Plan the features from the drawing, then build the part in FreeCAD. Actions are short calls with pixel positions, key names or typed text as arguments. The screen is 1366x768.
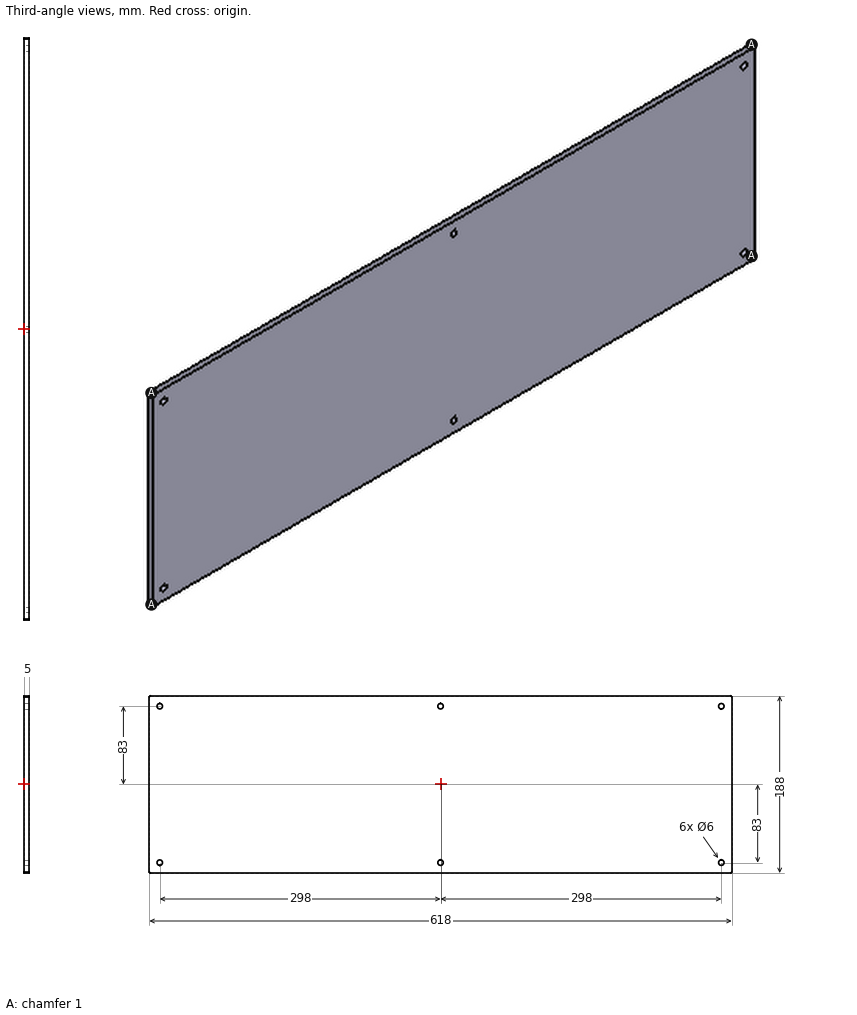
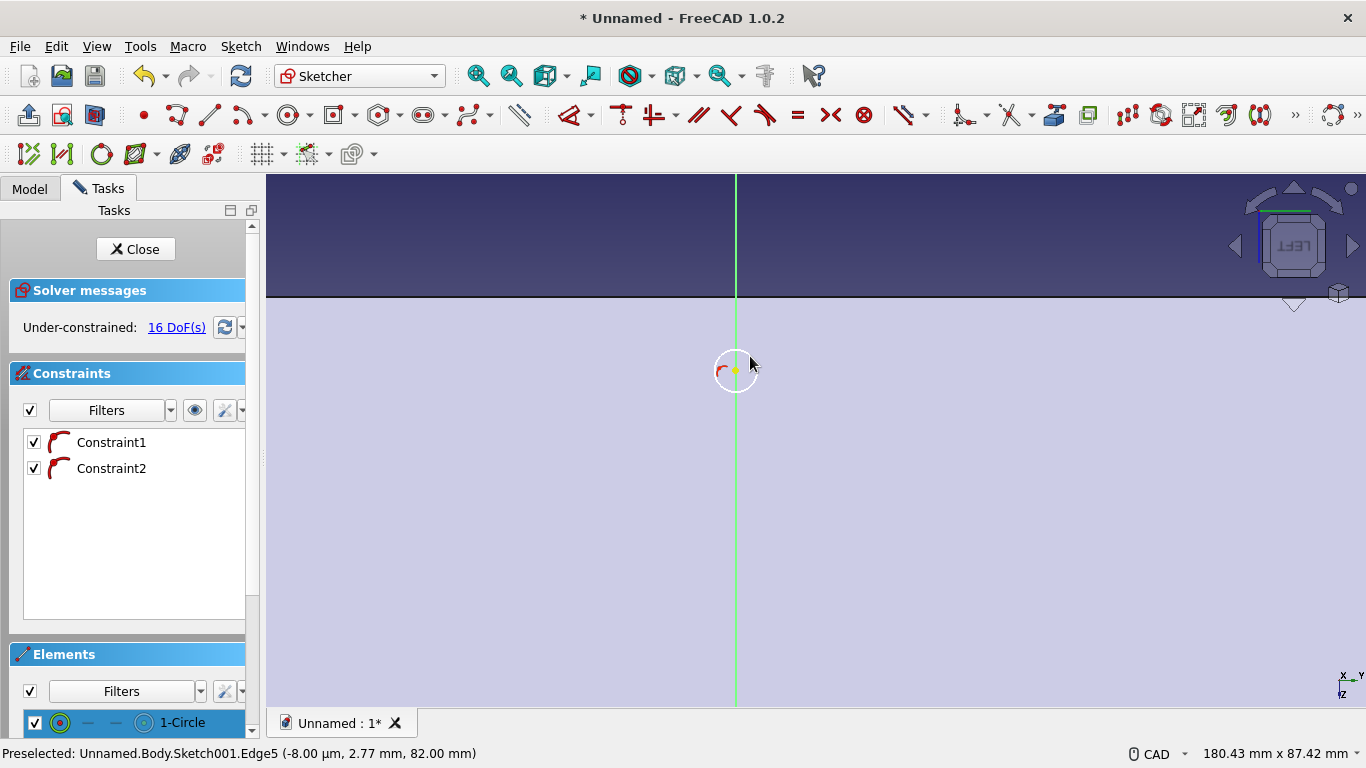
click(751, 356)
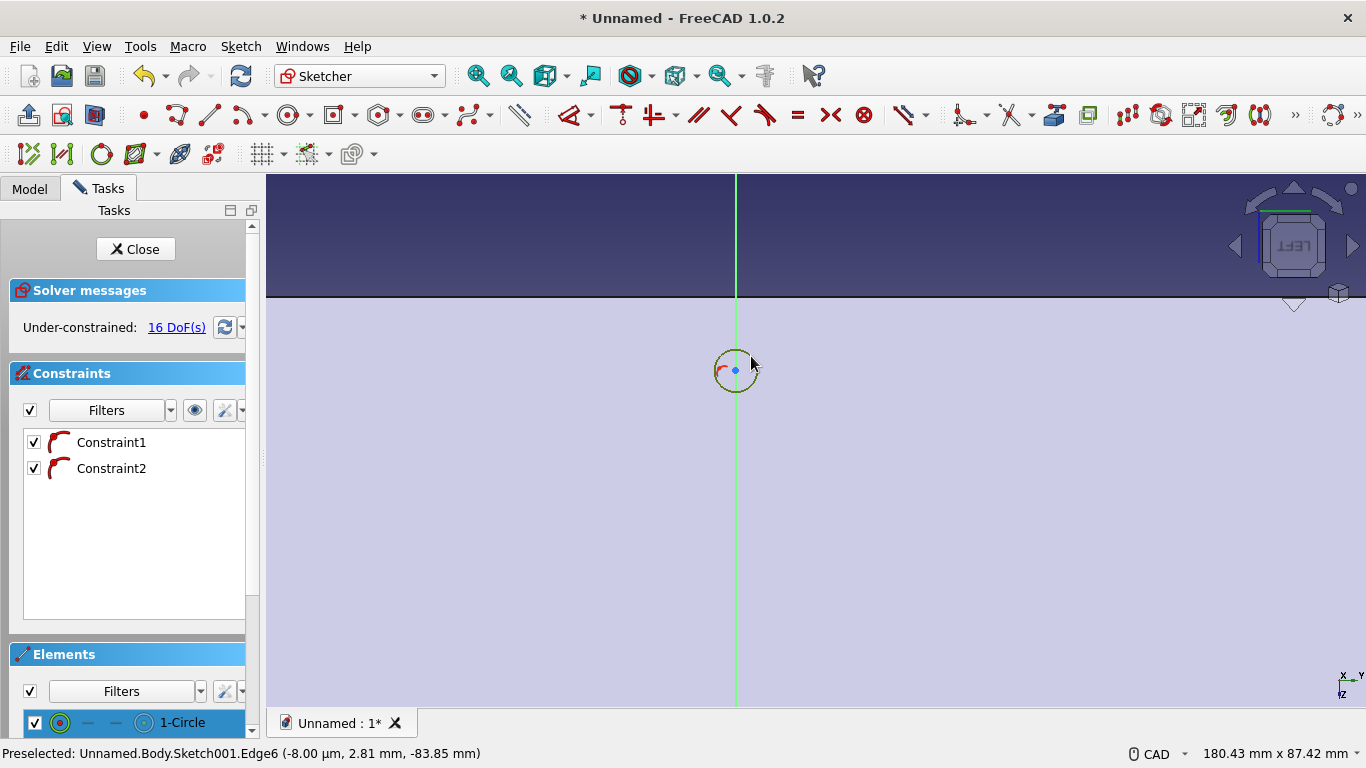
click(798, 116)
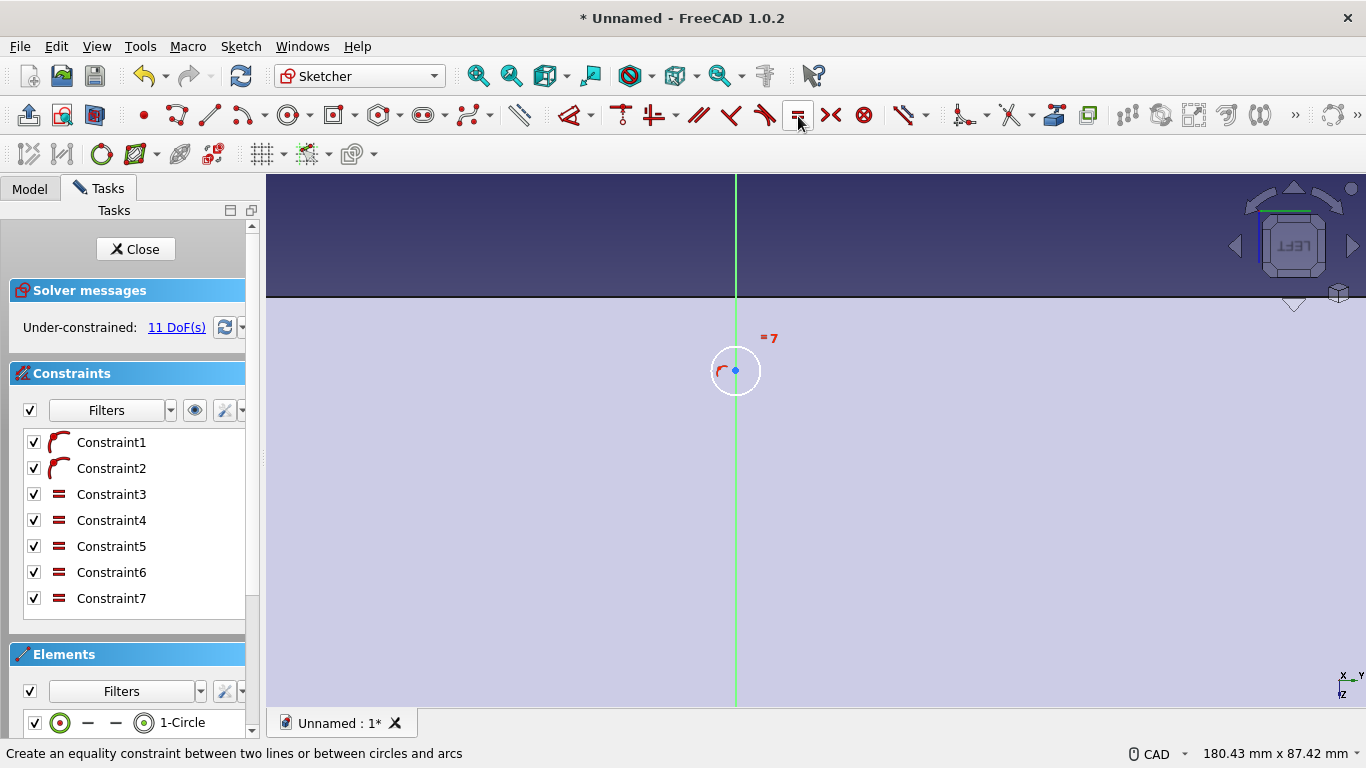
scroll(750, 356, down, 9)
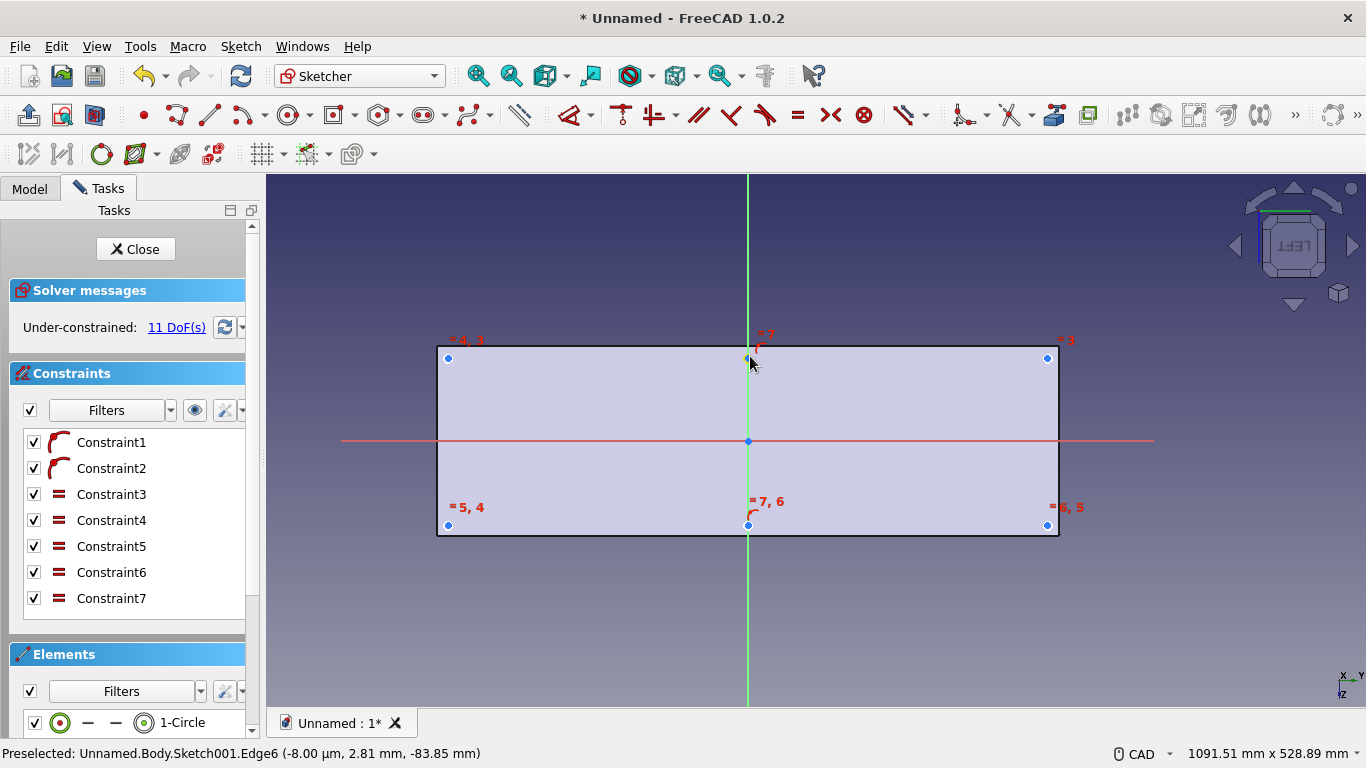
click(1048, 359)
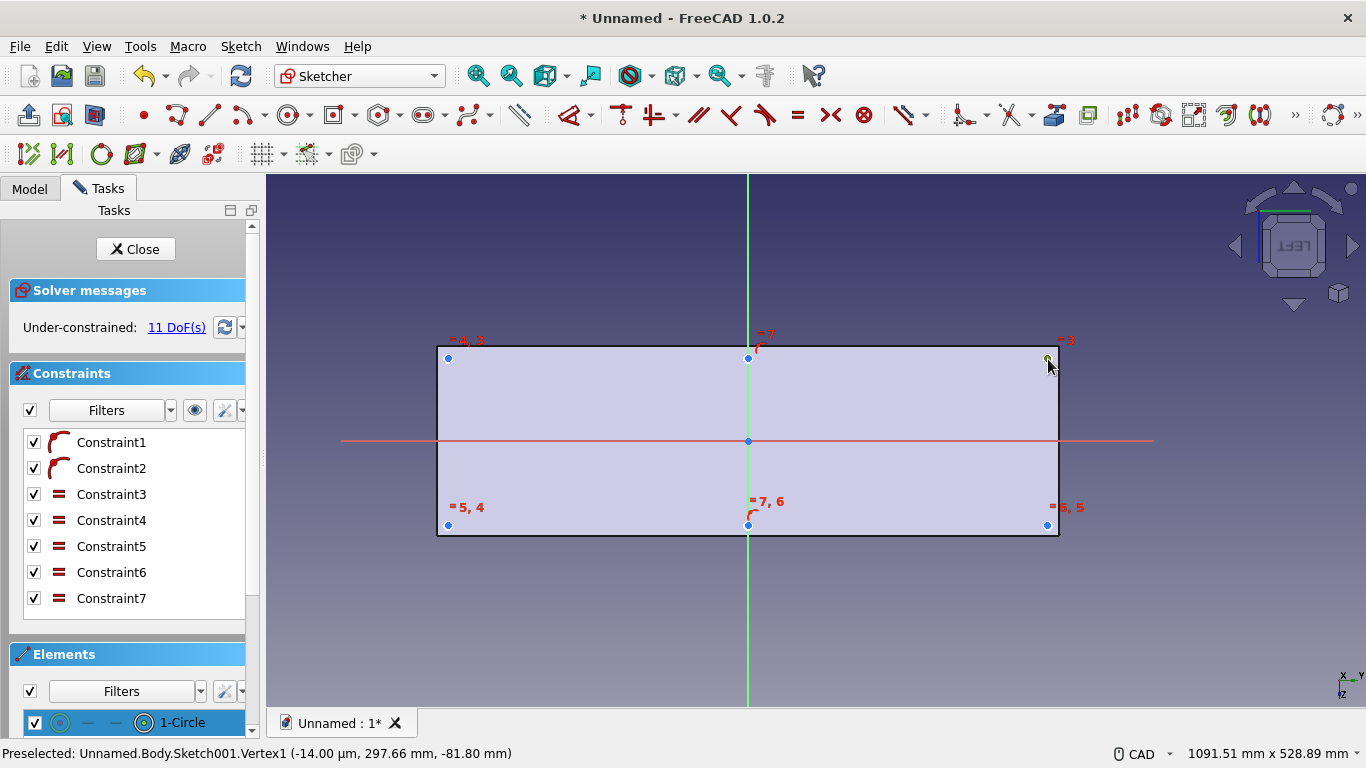
click(448, 359)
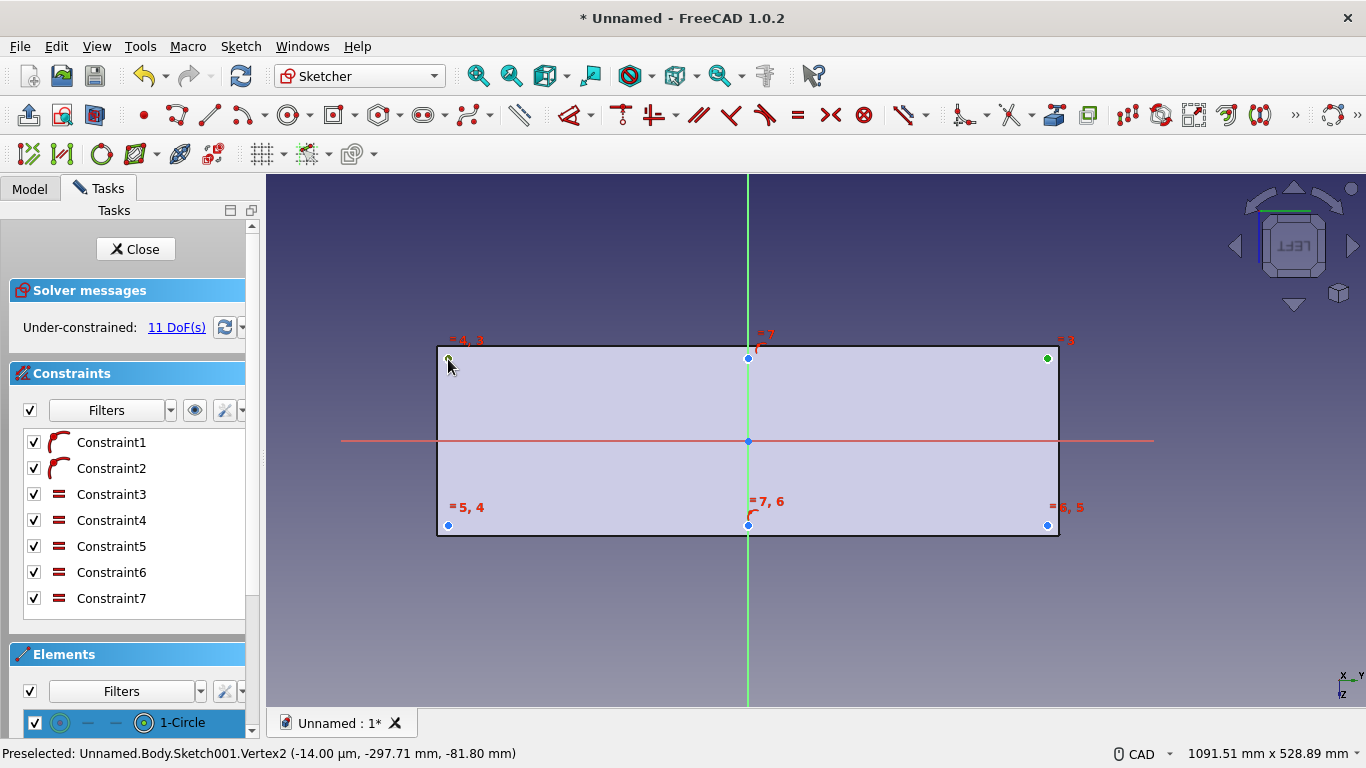
click(676, 116)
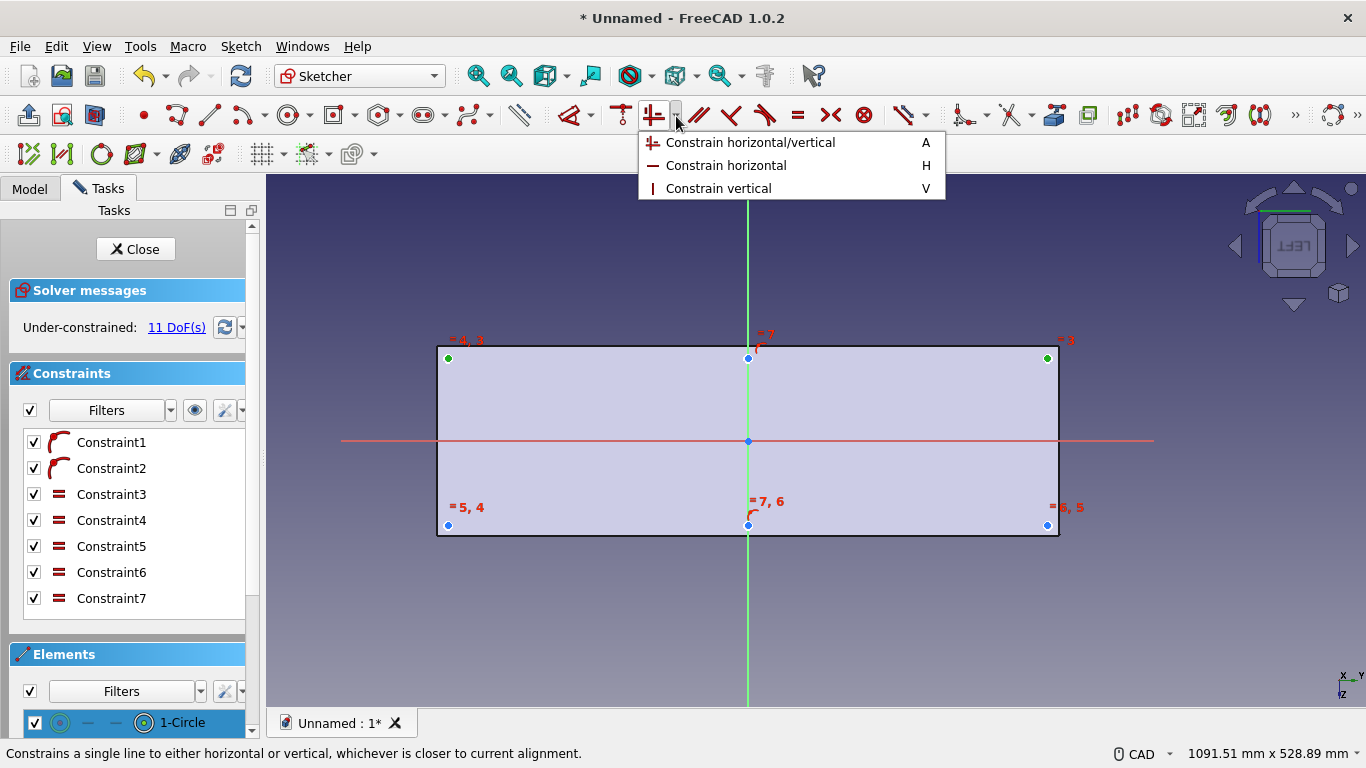
click(792, 166)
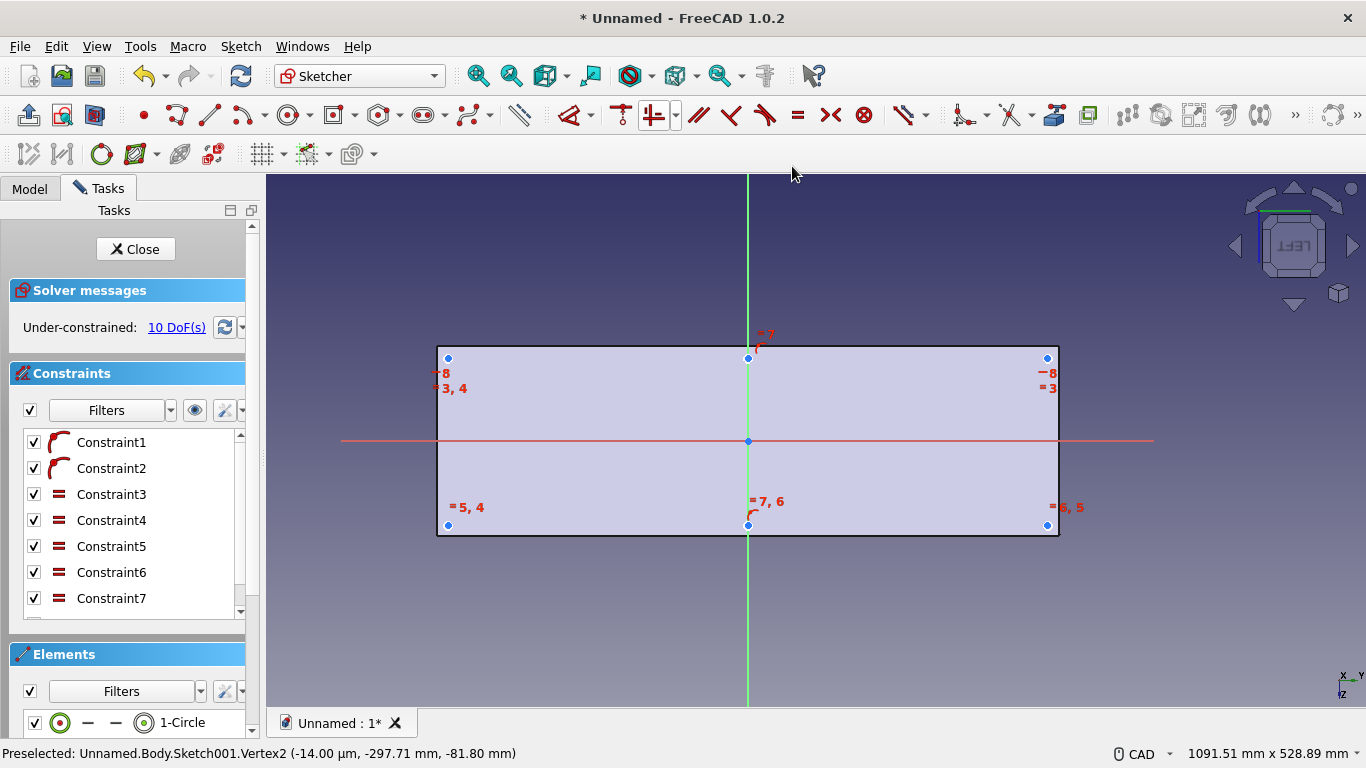
click(448, 359)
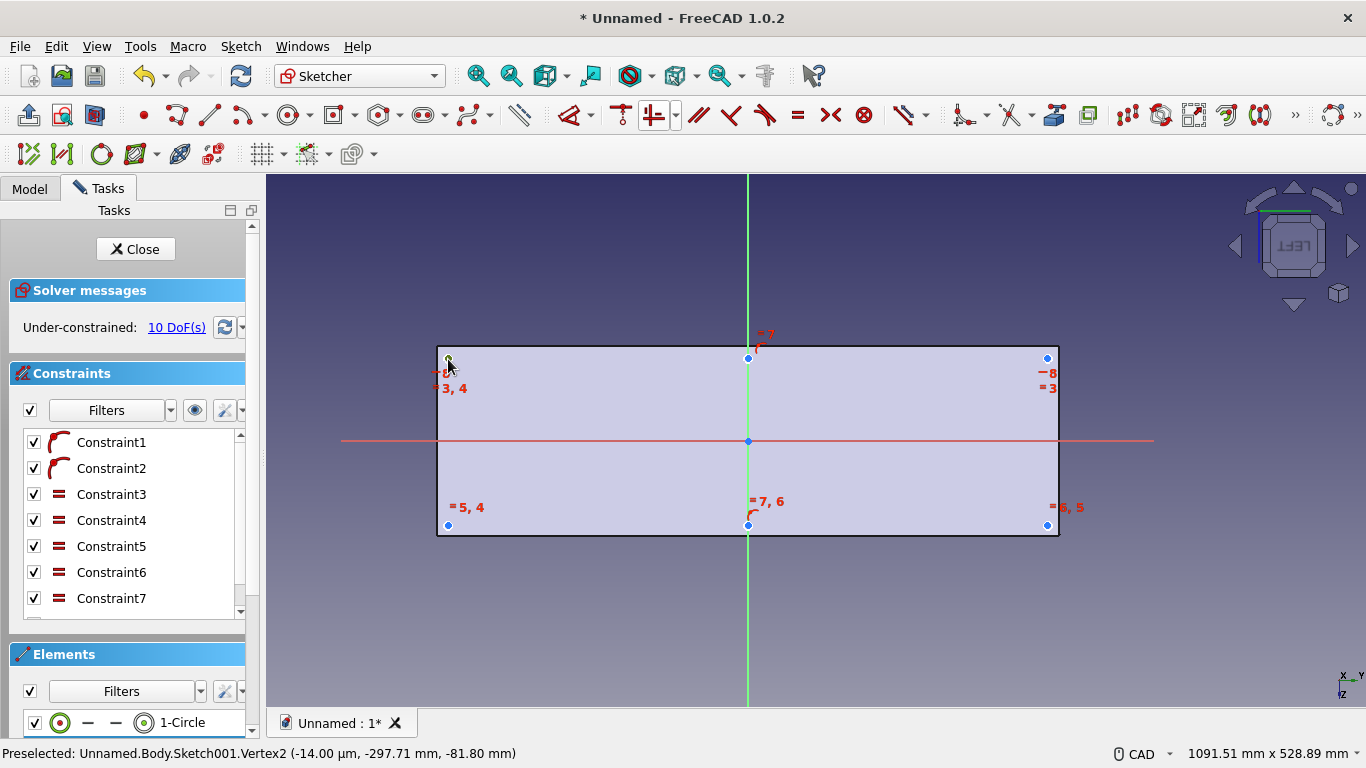
click(448, 526)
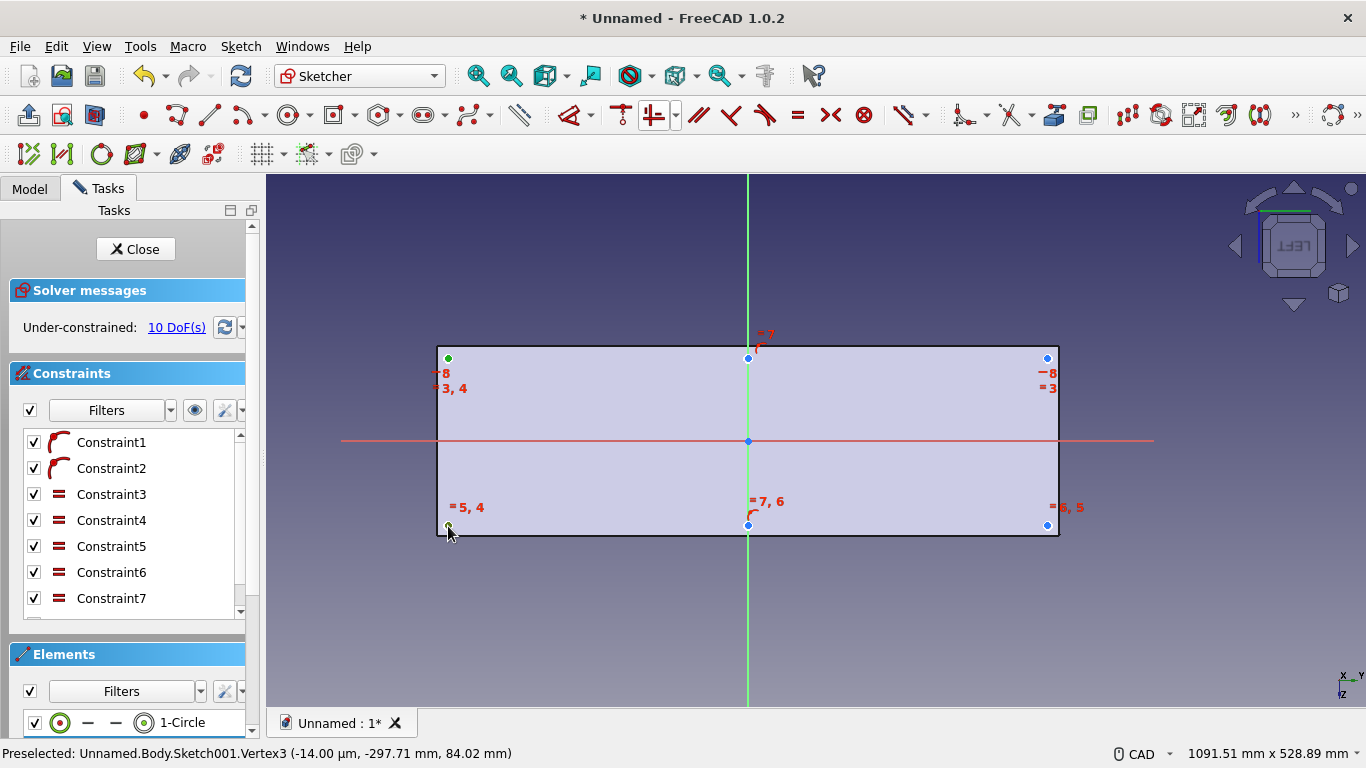
click(676, 116)